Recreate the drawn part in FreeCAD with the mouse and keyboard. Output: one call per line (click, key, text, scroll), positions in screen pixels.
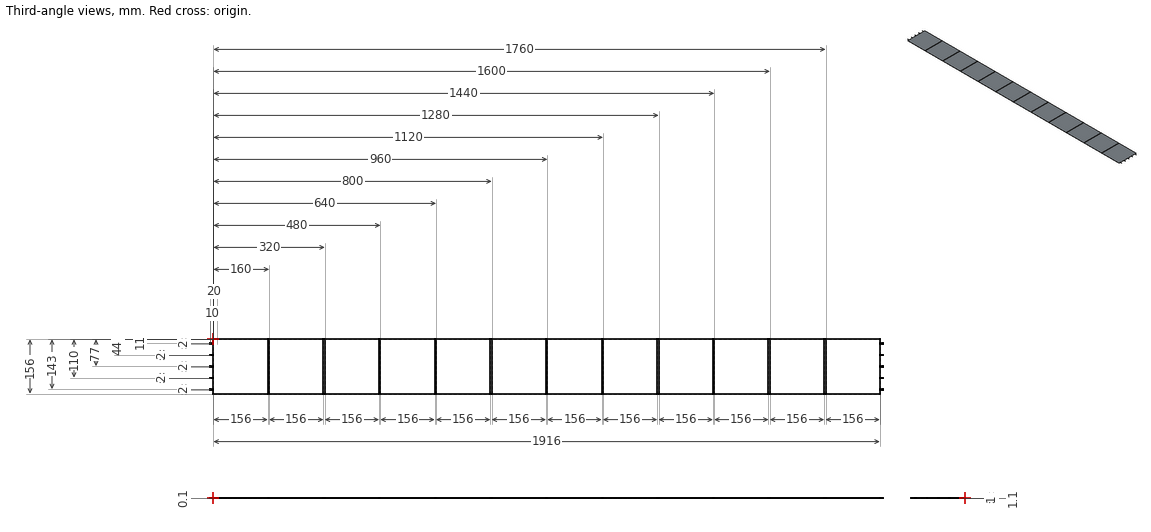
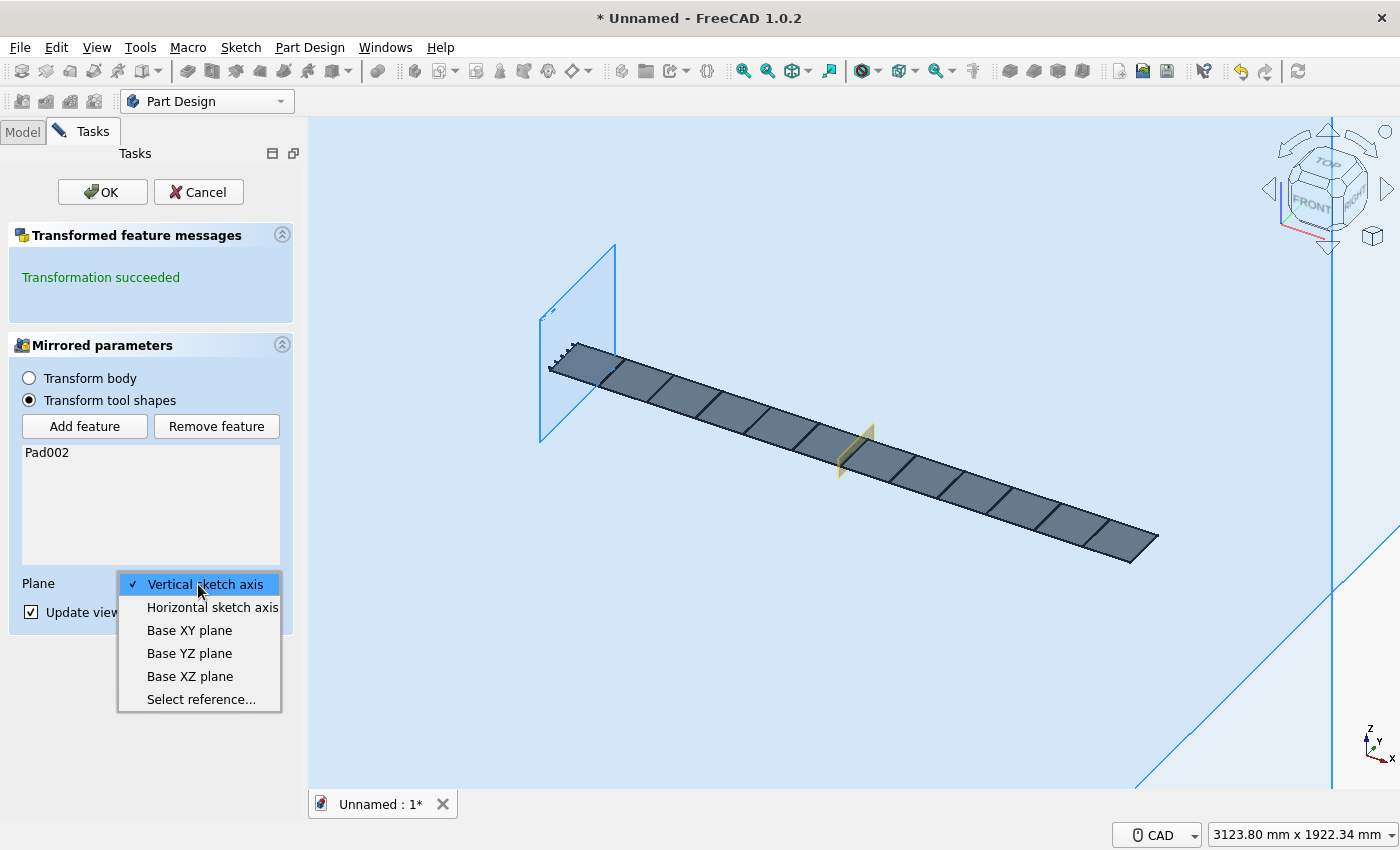
click(198, 700)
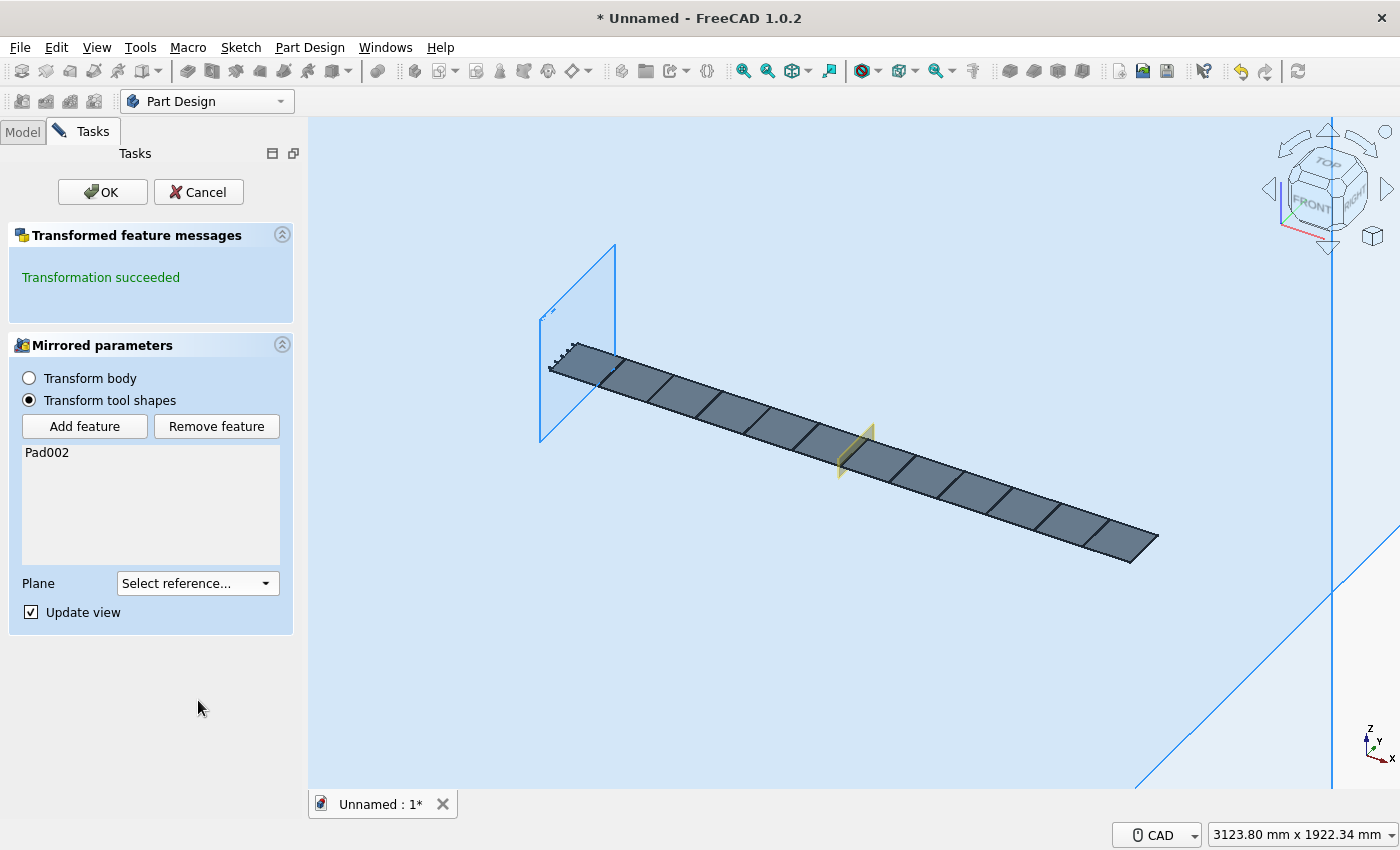
click(23, 131)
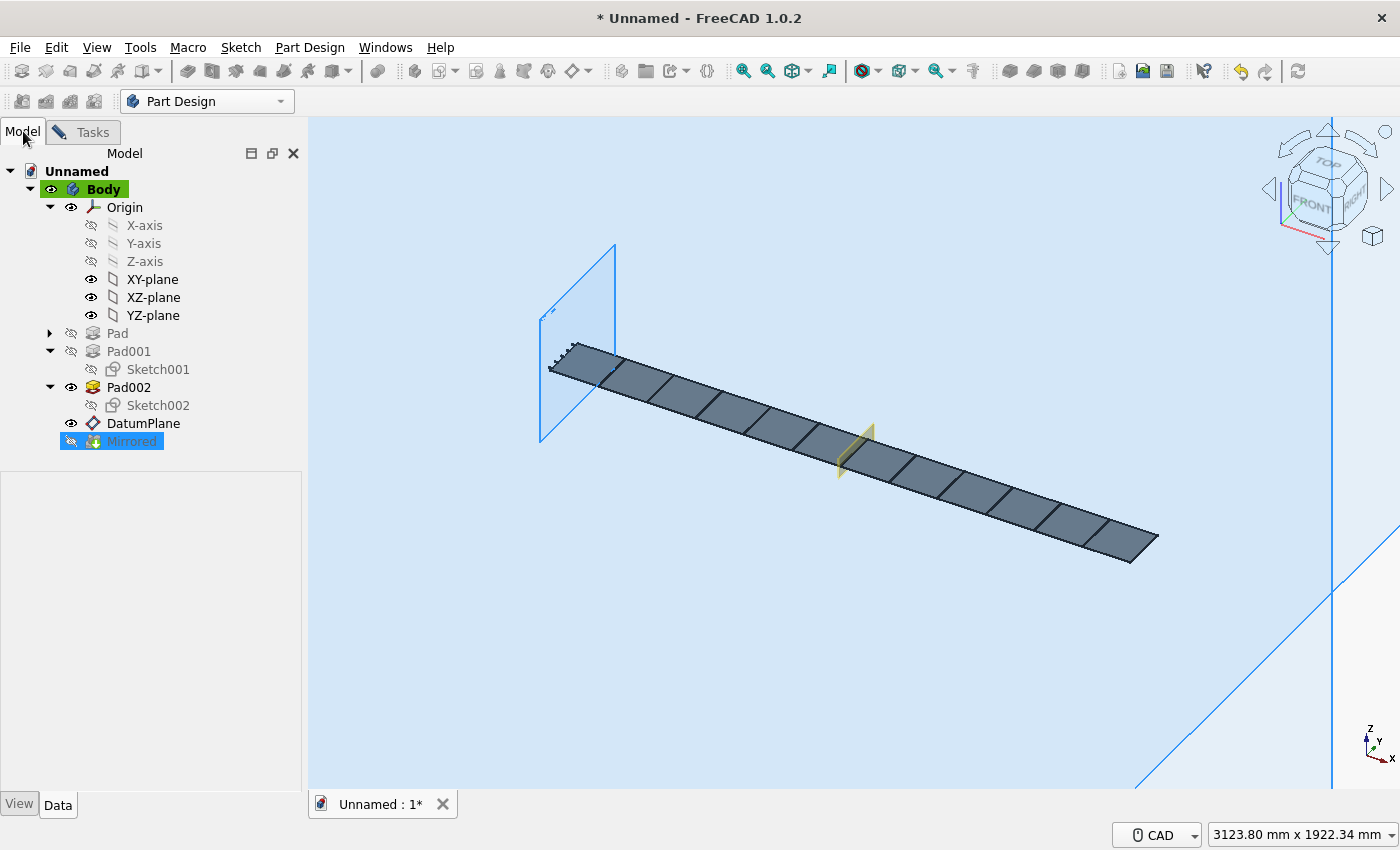
click(116, 423)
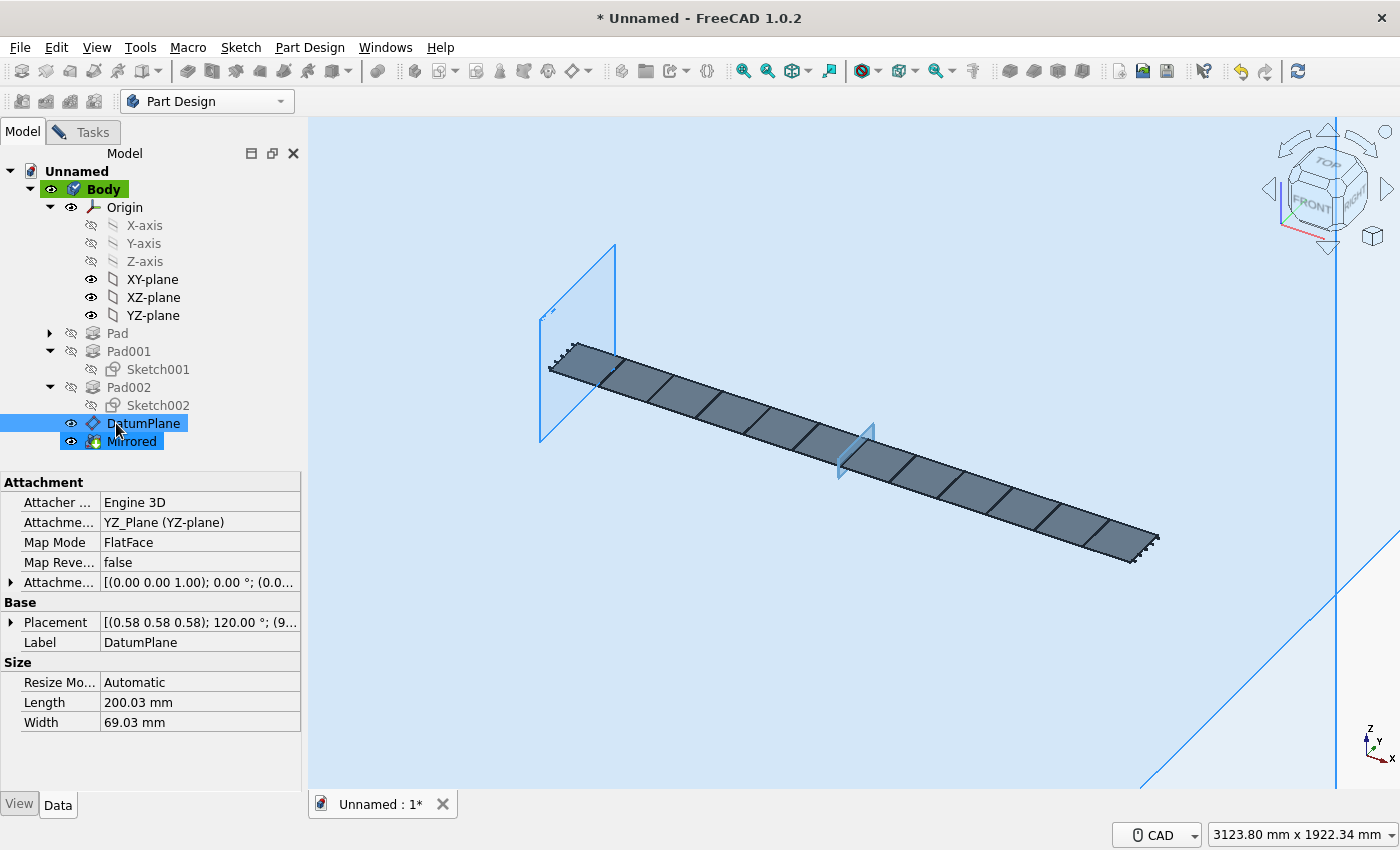
click(84, 131)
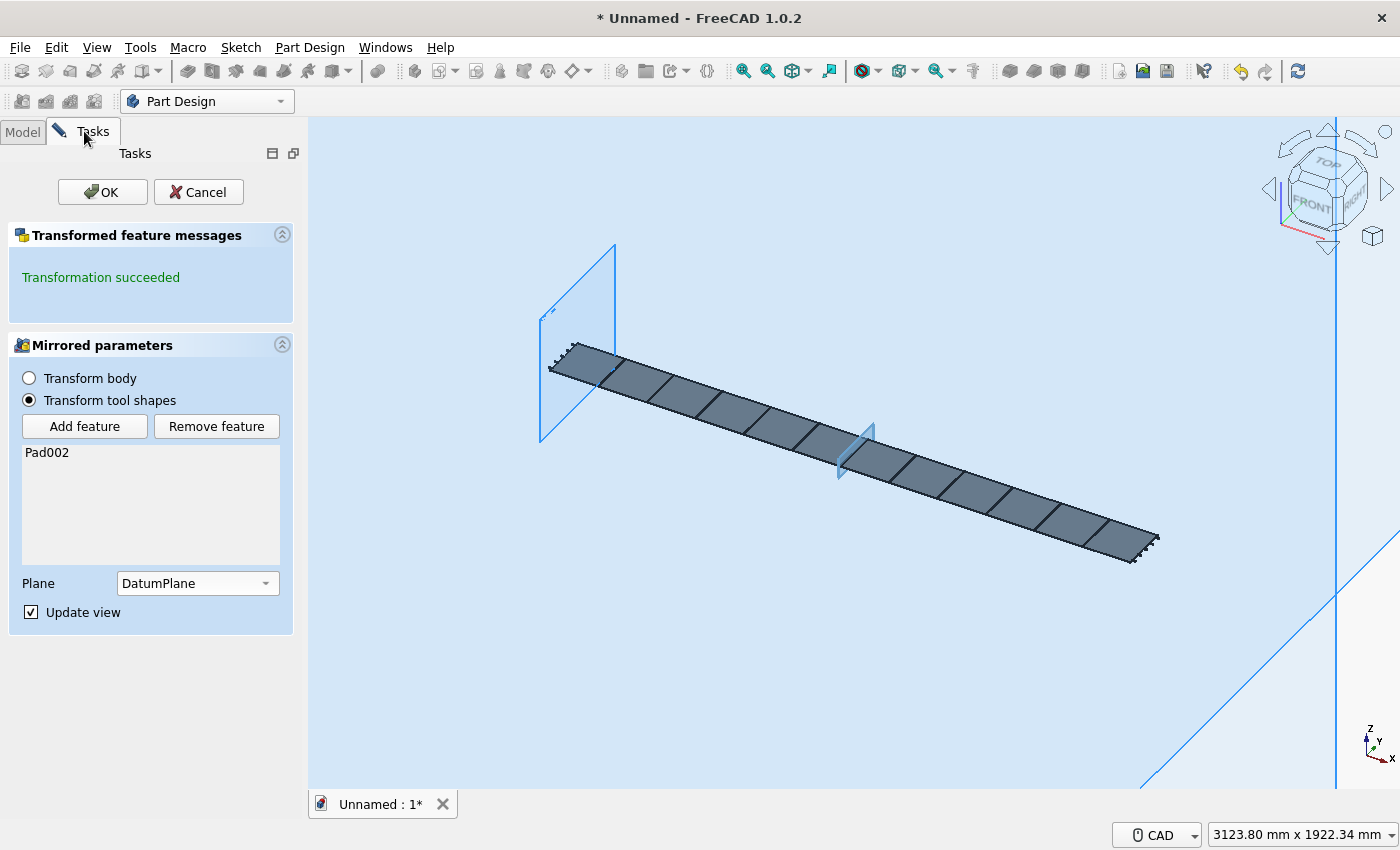
click(103, 192)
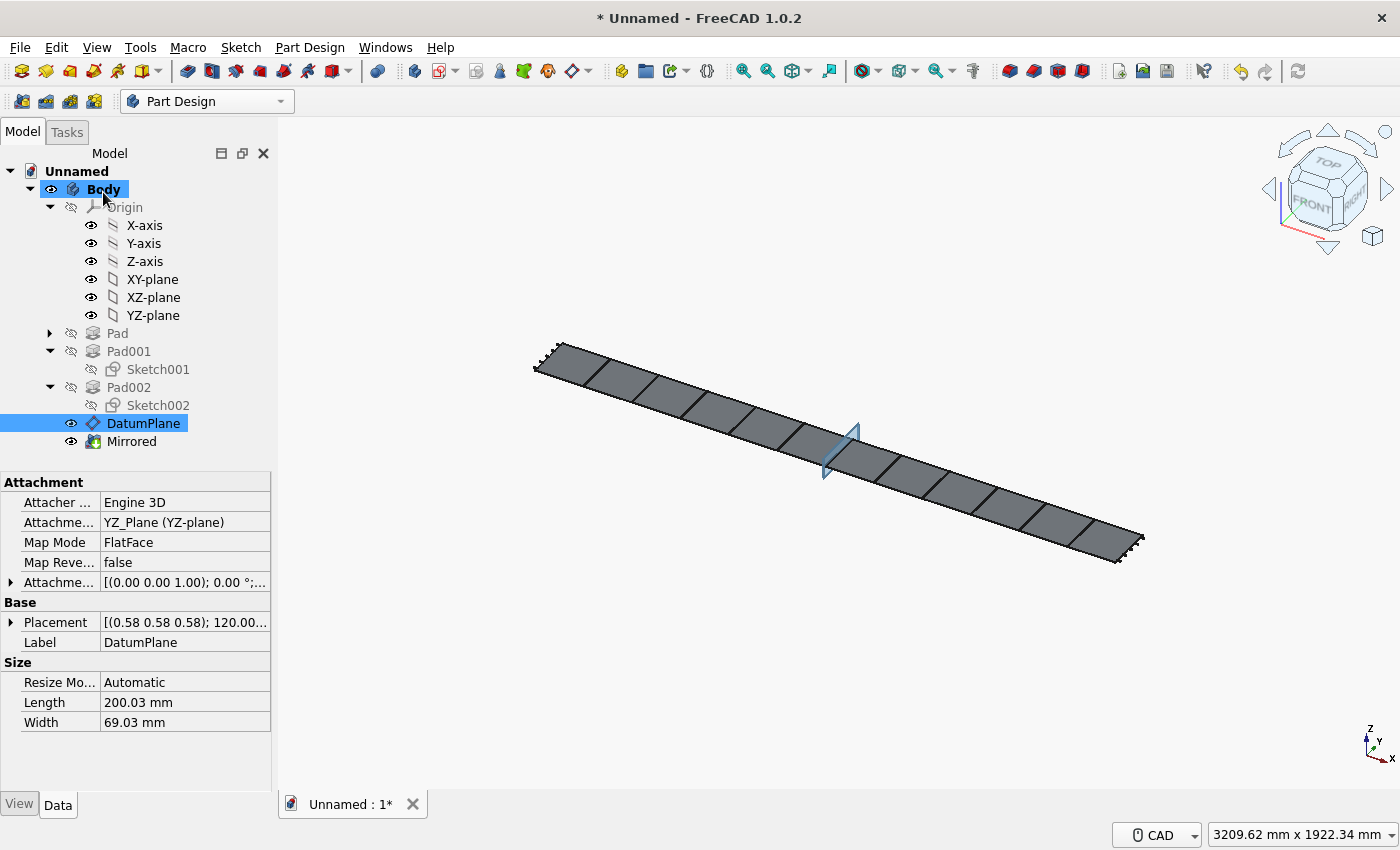
click(116, 423)
key(space)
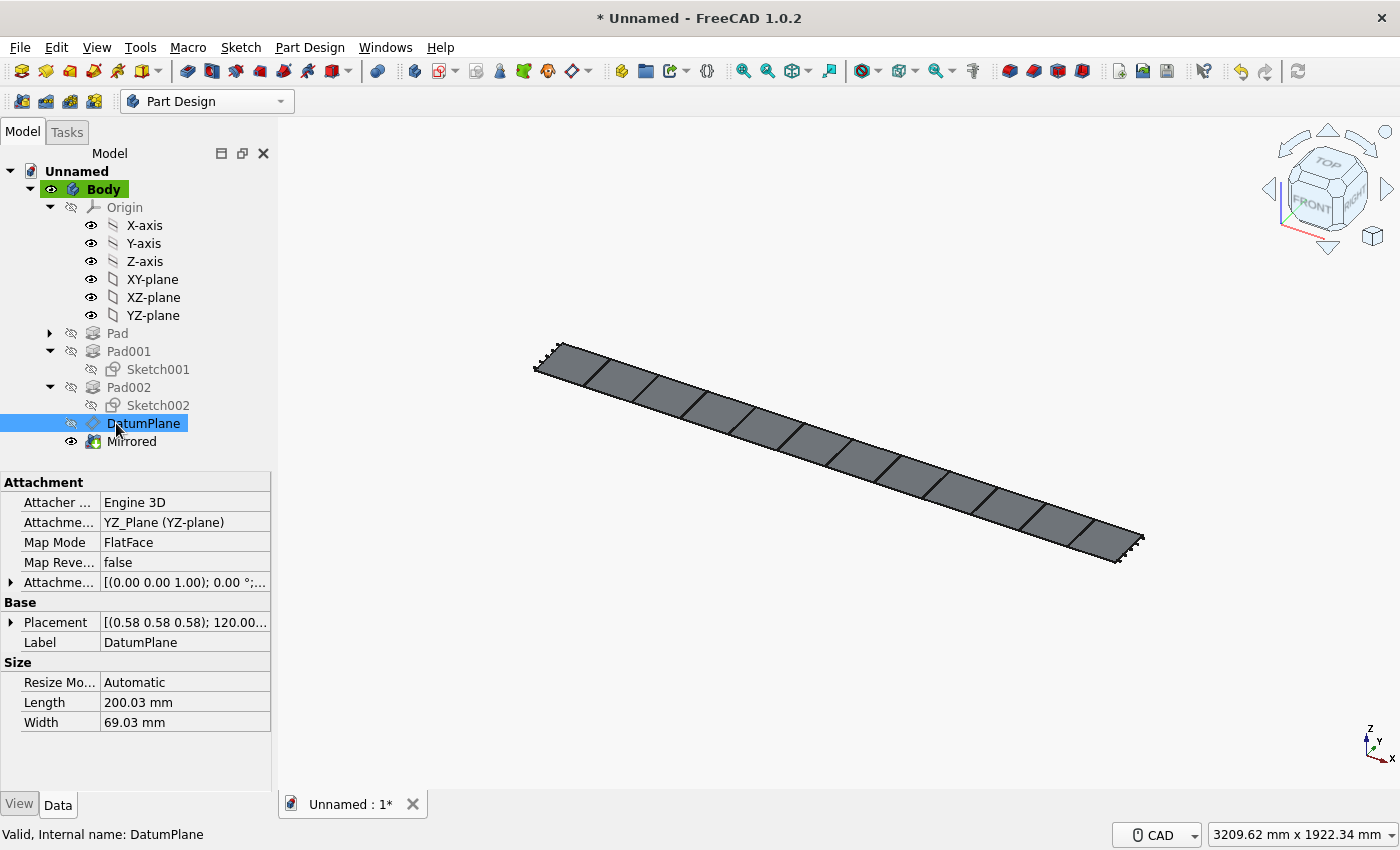
key(0)